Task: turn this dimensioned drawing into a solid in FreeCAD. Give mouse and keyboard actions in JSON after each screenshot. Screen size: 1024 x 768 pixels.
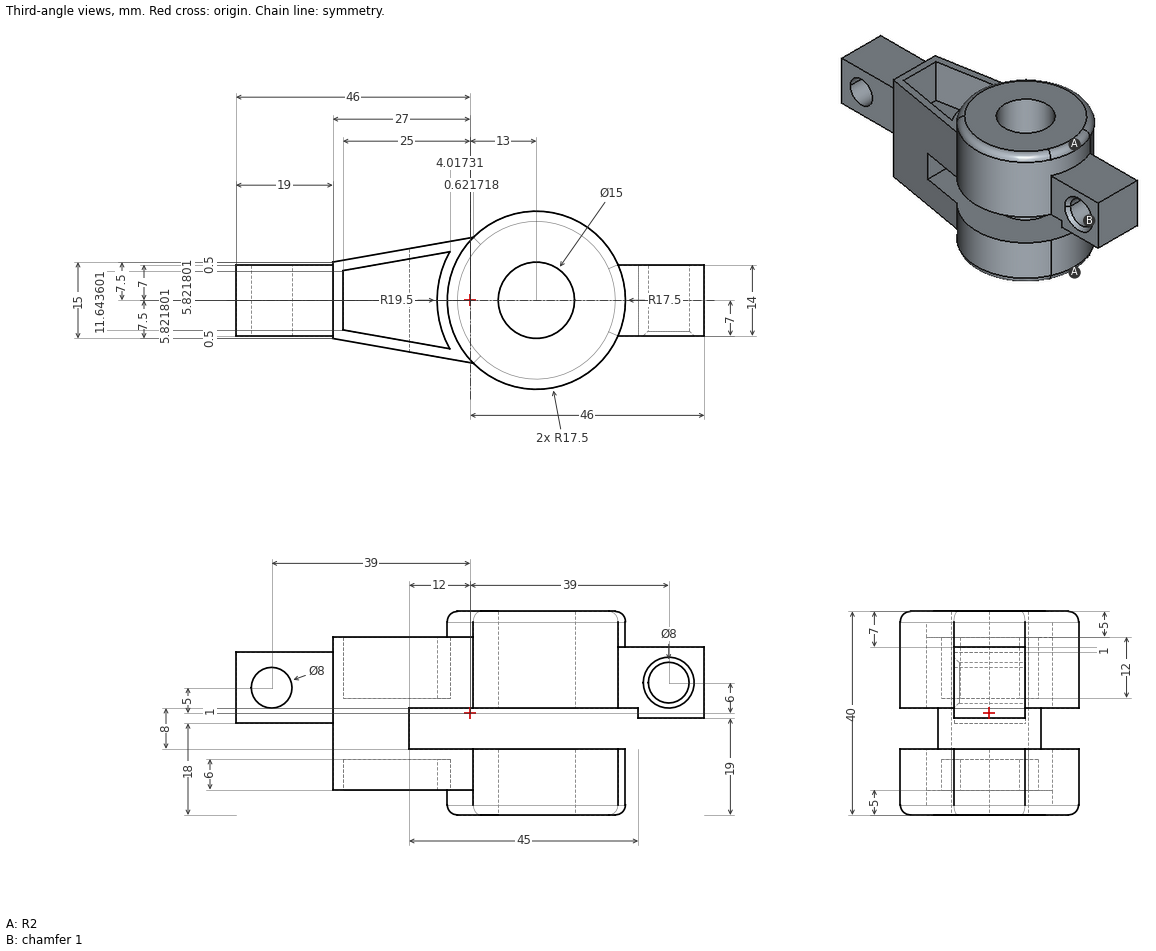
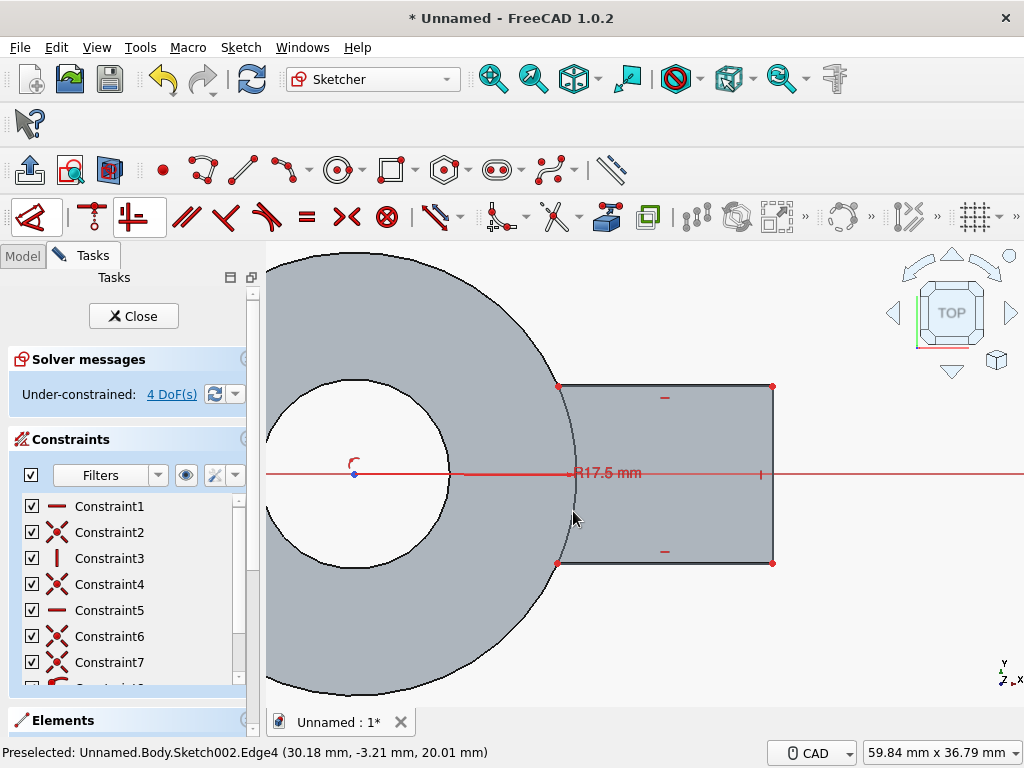
{"action": "left_click", "coordinate": [773, 510]}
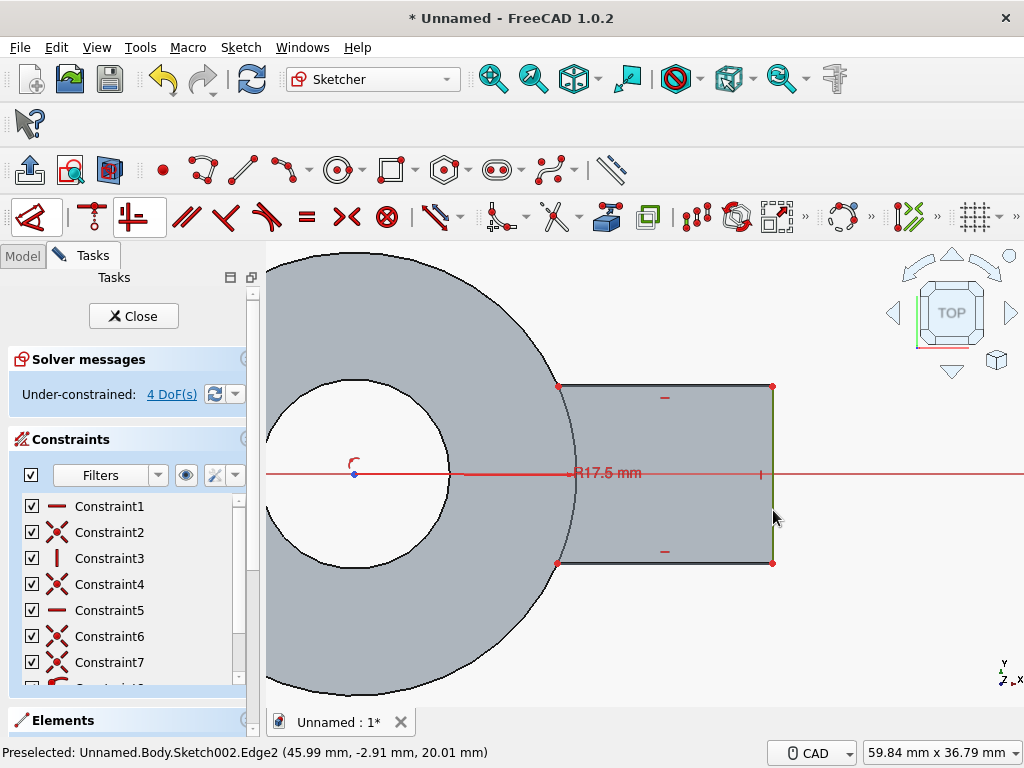
{"action": "left_click", "coordinate": [56, 218]}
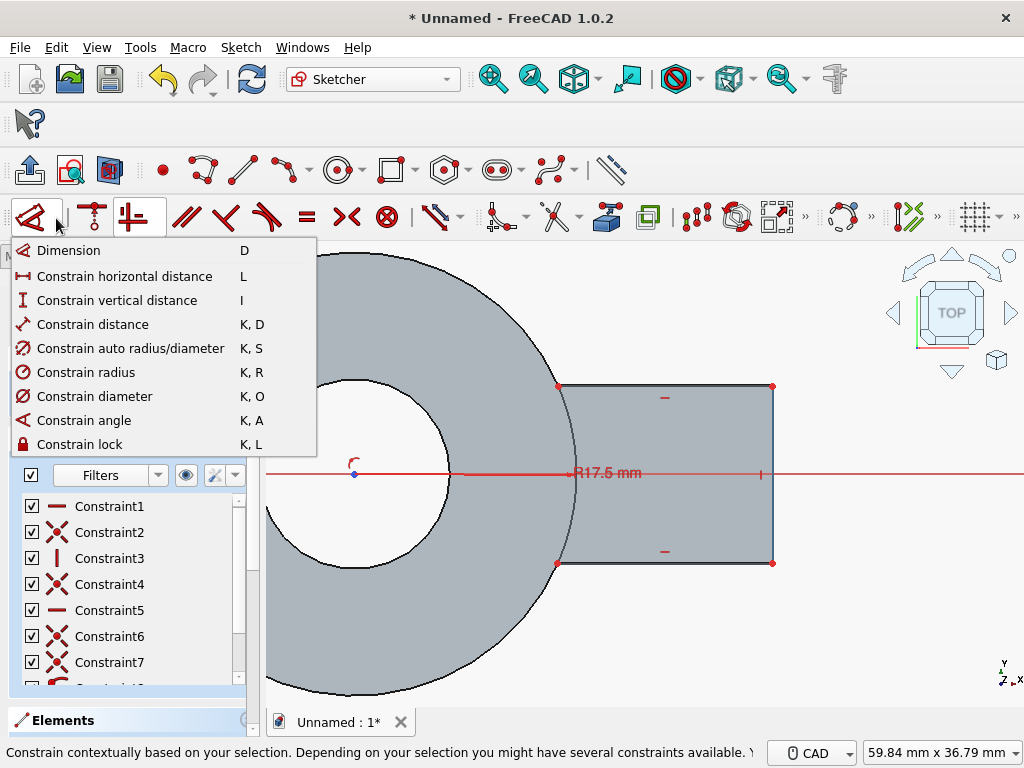
{"action": "left_click", "coordinate": [164, 300]}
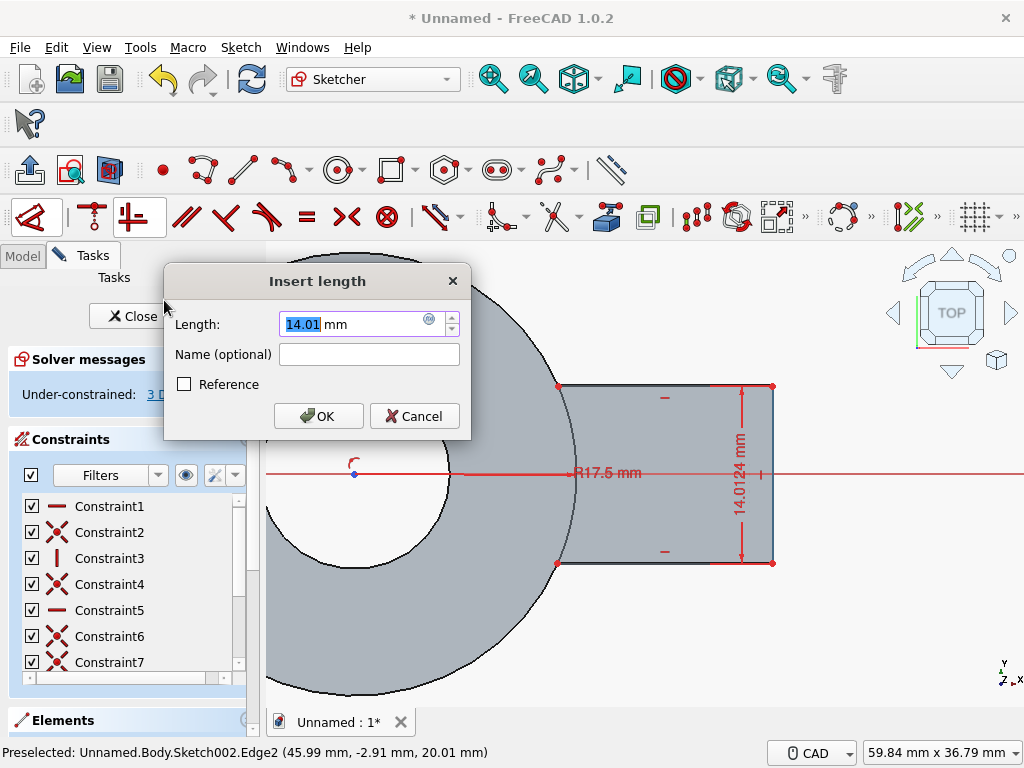
{"action": "type", "text": "14"}
{"action": "key", "text": "Return"}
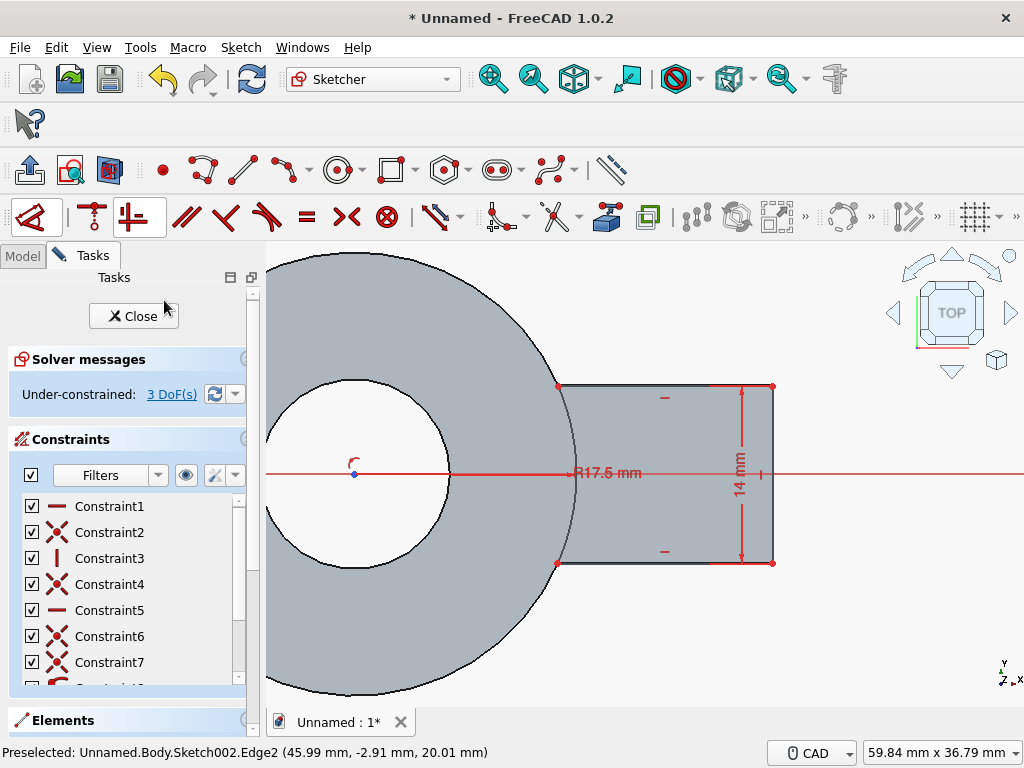
{"action": "left_click", "coordinate": [558, 564]}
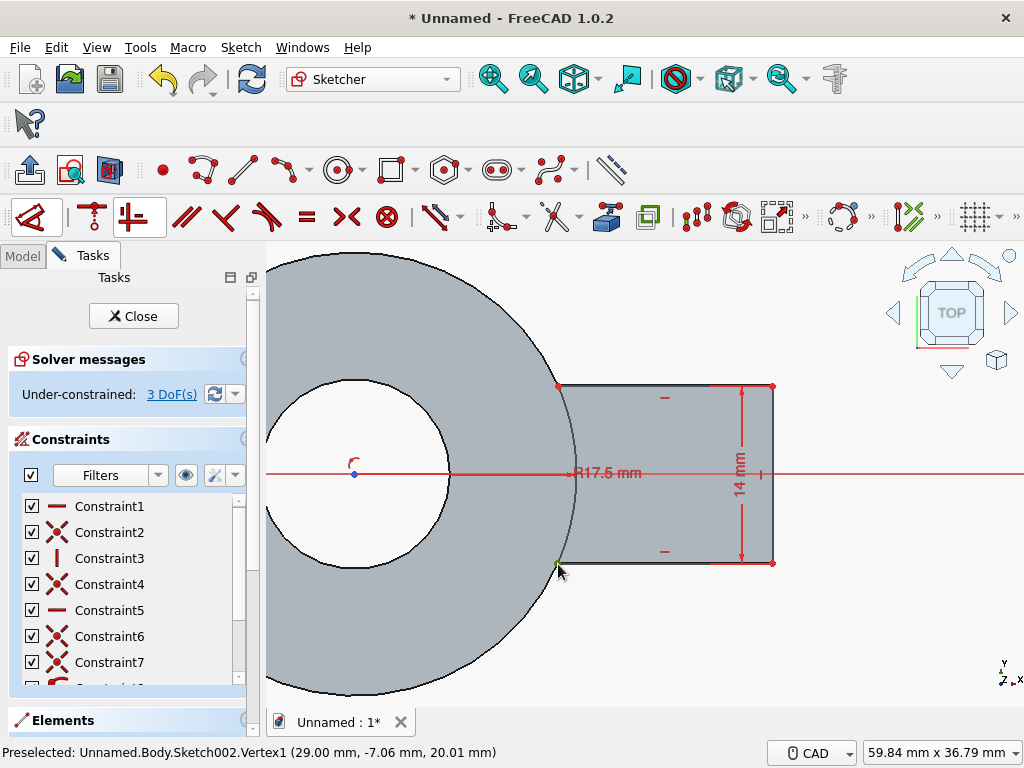
{"action": "left_click", "coordinate": [56, 218]}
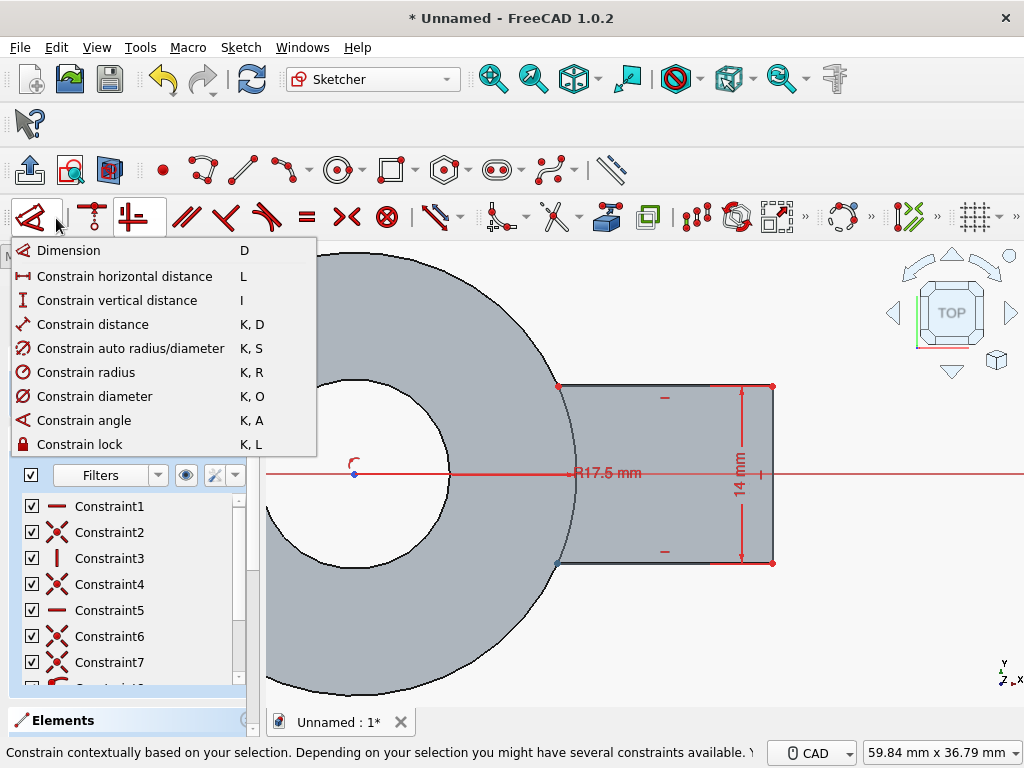
{"action": "left_click", "coordinate": [164, 300]}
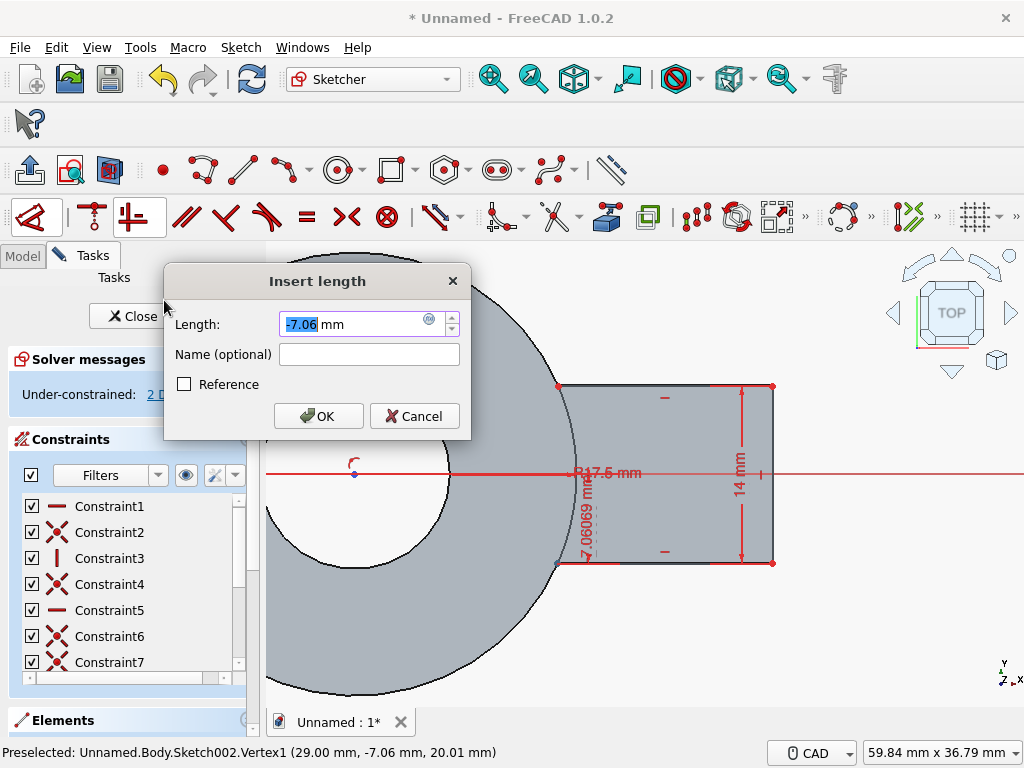
{"action": "type", "text": "-7"}
{"action": "key", "text": "Return"}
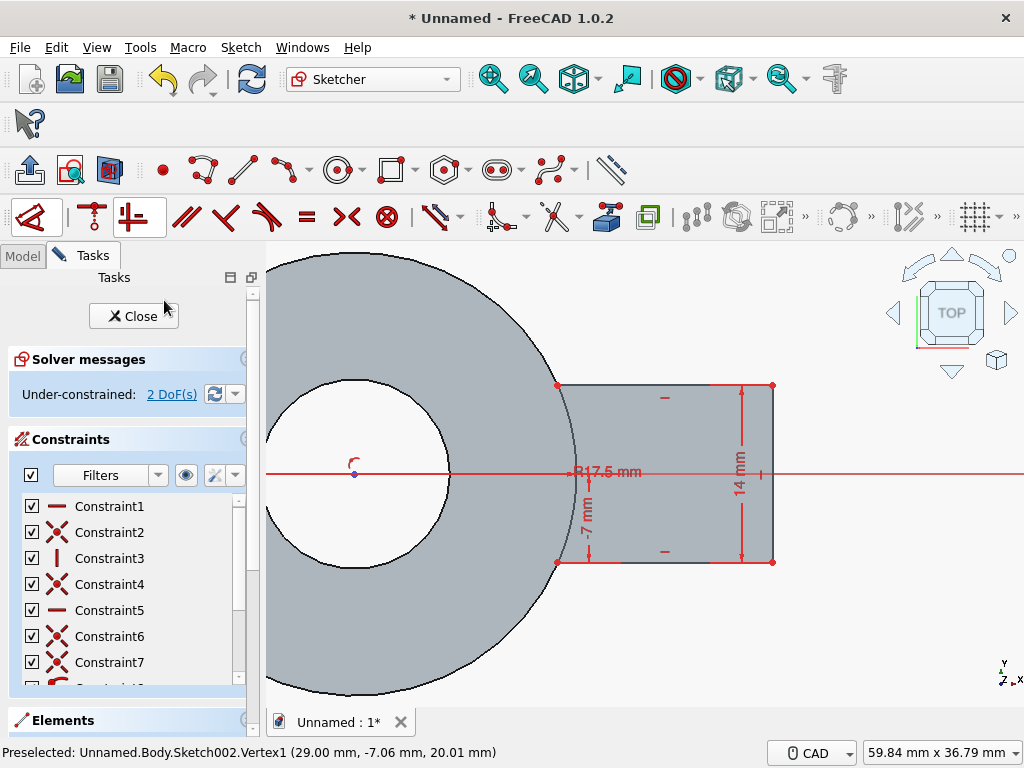
{"action": "left_click", "coordinate": [773, 563]}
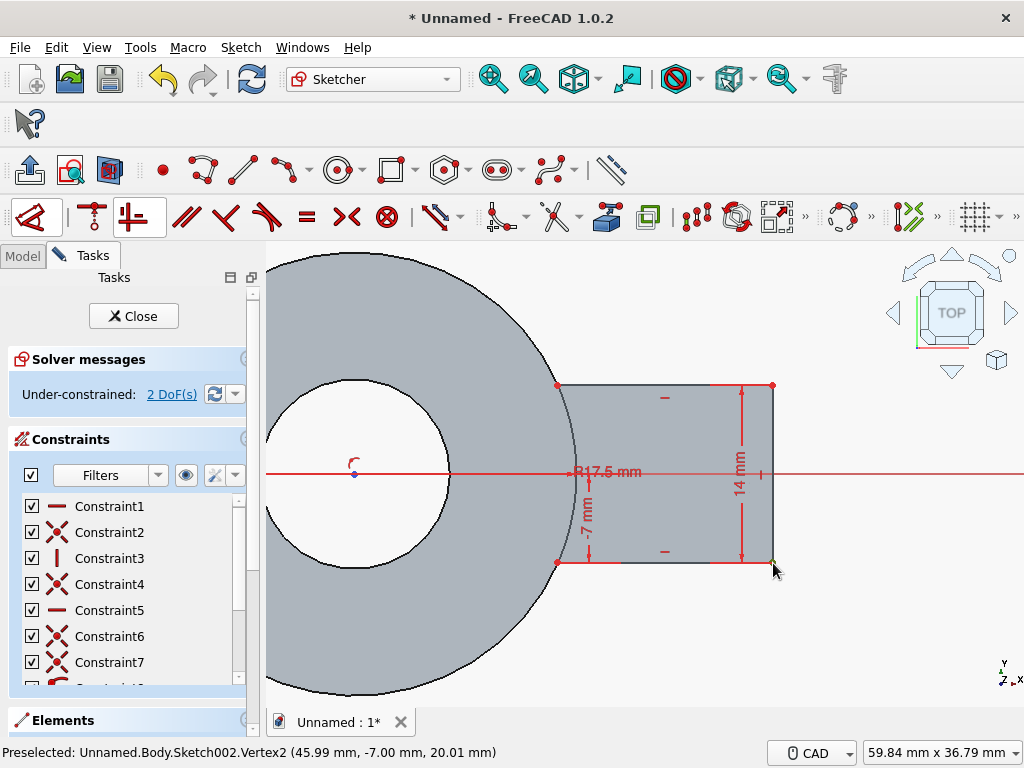
{"action": "left_click", "coordinate": [56, 218]}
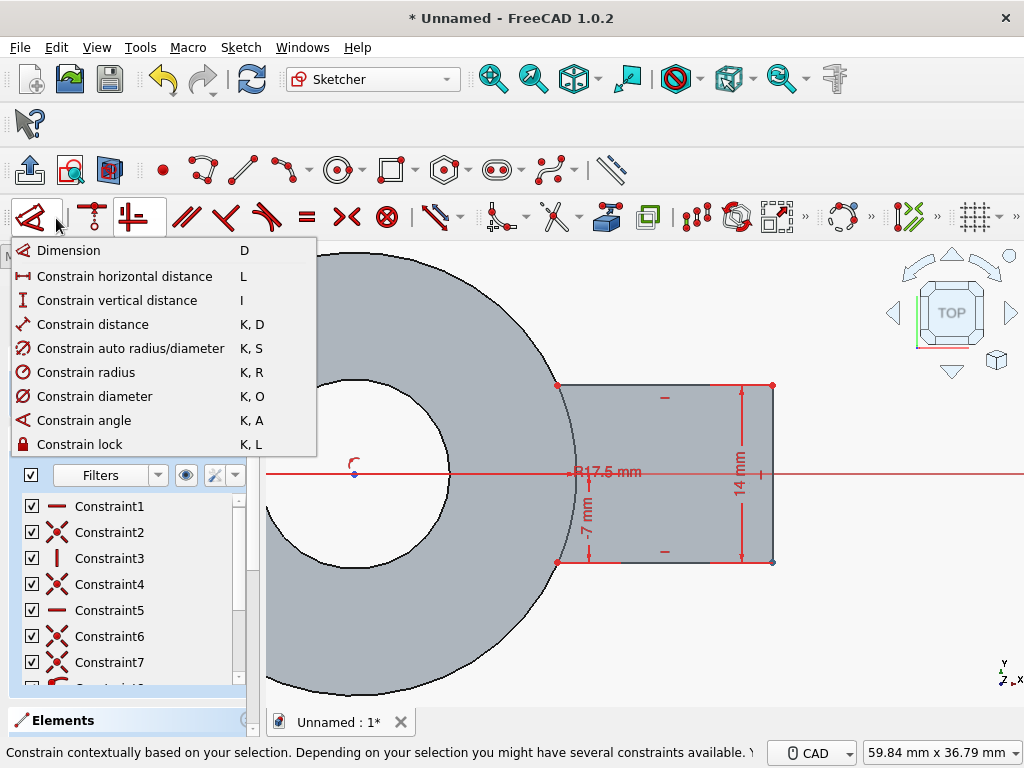
{"action": "left_click", "coordinate": [164, 276]}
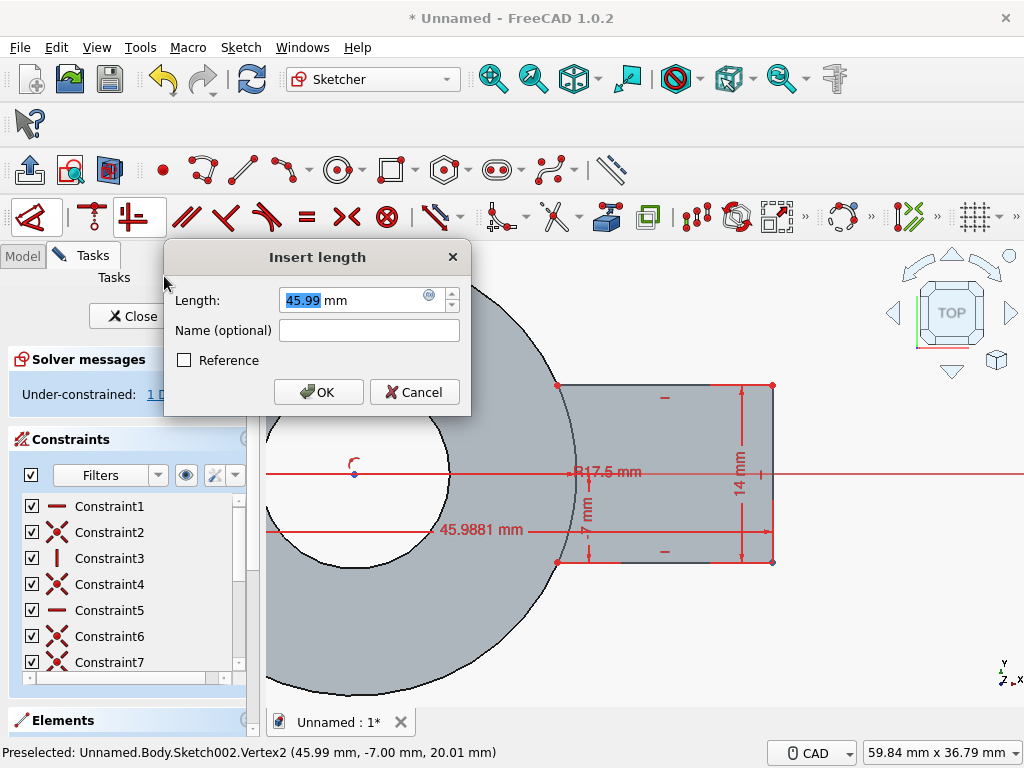
{"action": "type", "text": "46"}
{"action": "key", "text": "Return"}